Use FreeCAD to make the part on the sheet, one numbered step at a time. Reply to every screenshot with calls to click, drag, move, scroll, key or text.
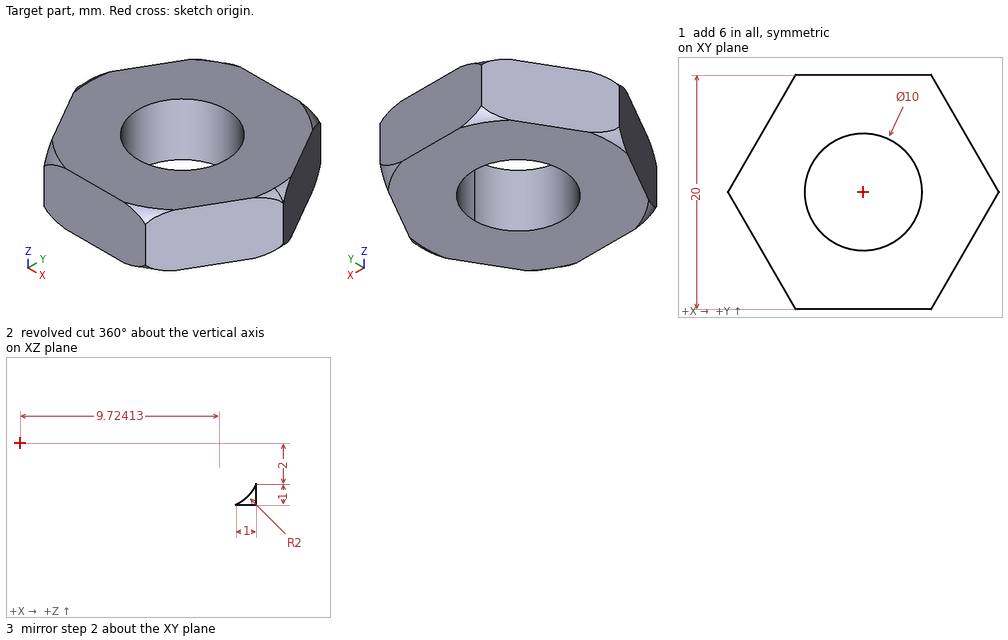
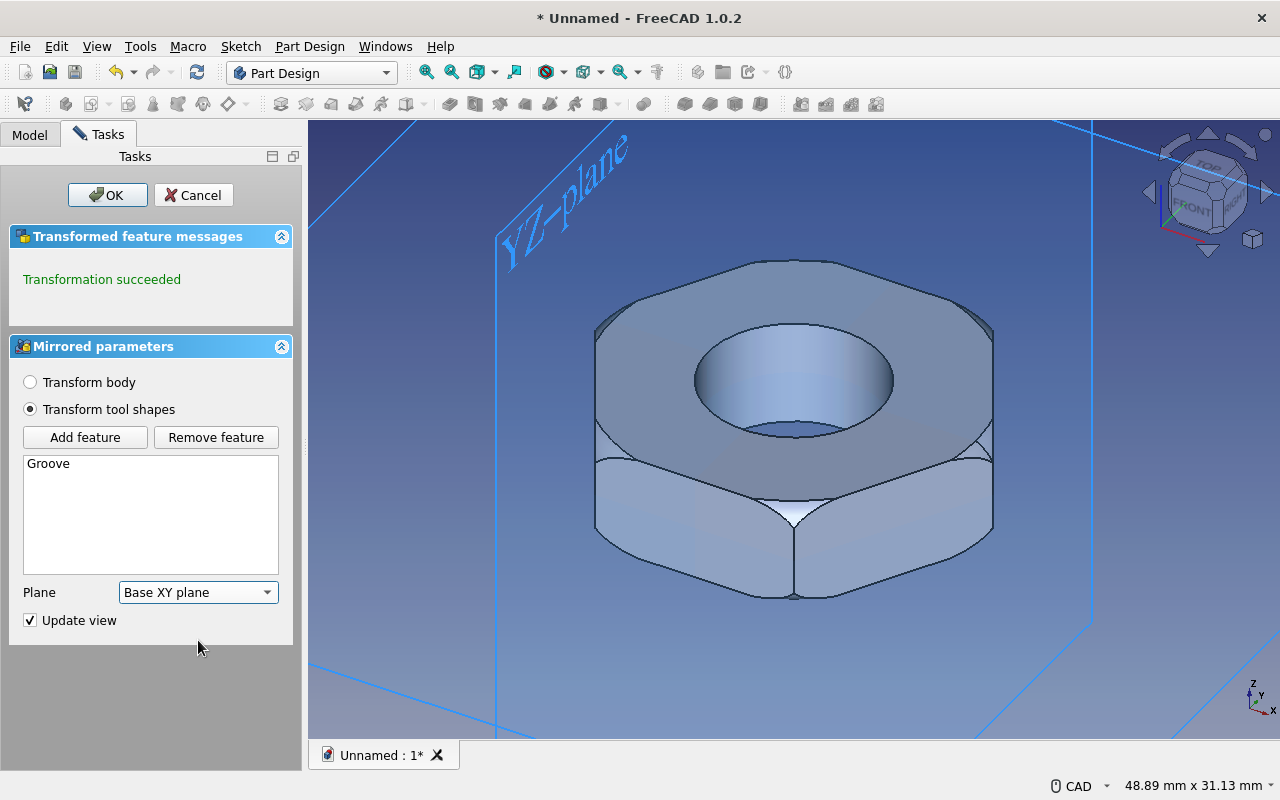
click(108, 195)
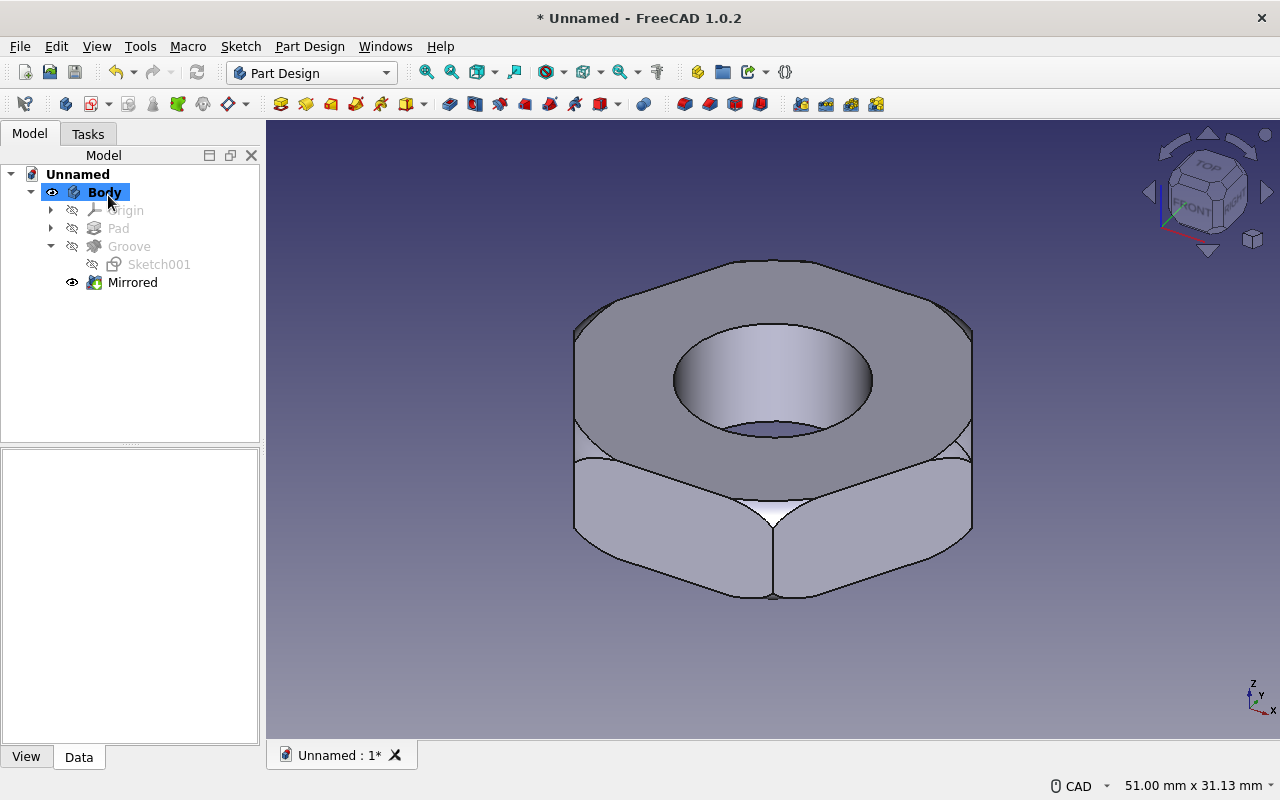
key(0)